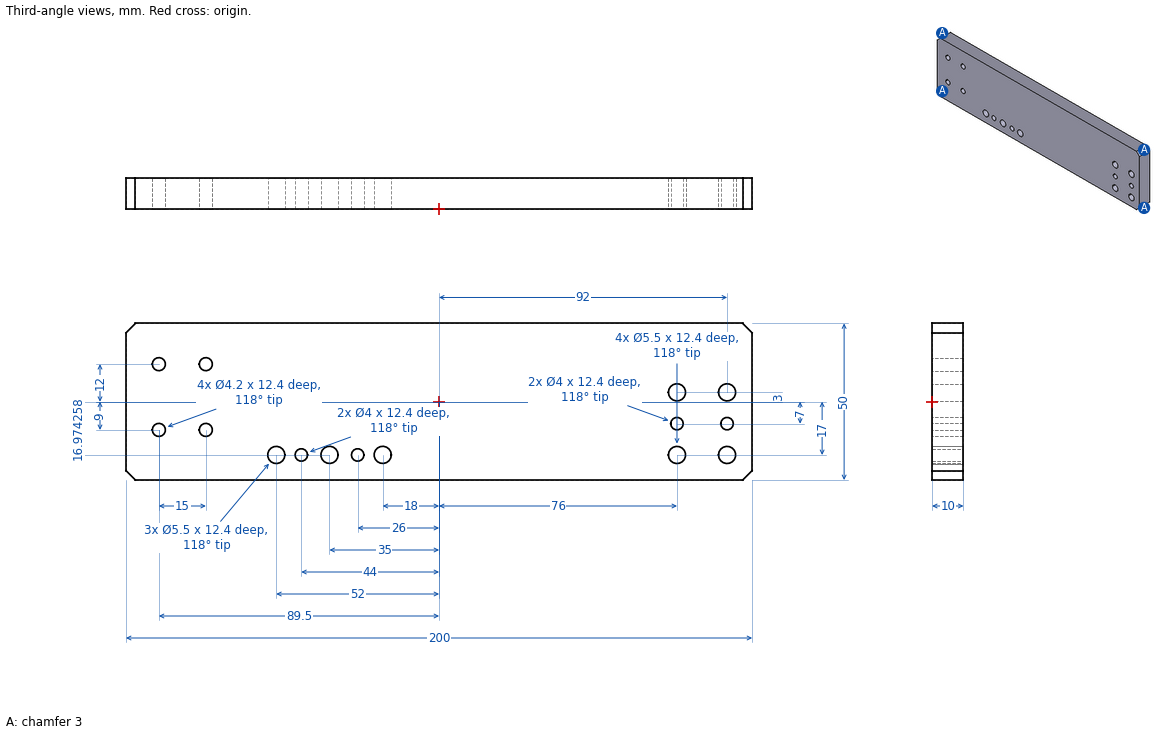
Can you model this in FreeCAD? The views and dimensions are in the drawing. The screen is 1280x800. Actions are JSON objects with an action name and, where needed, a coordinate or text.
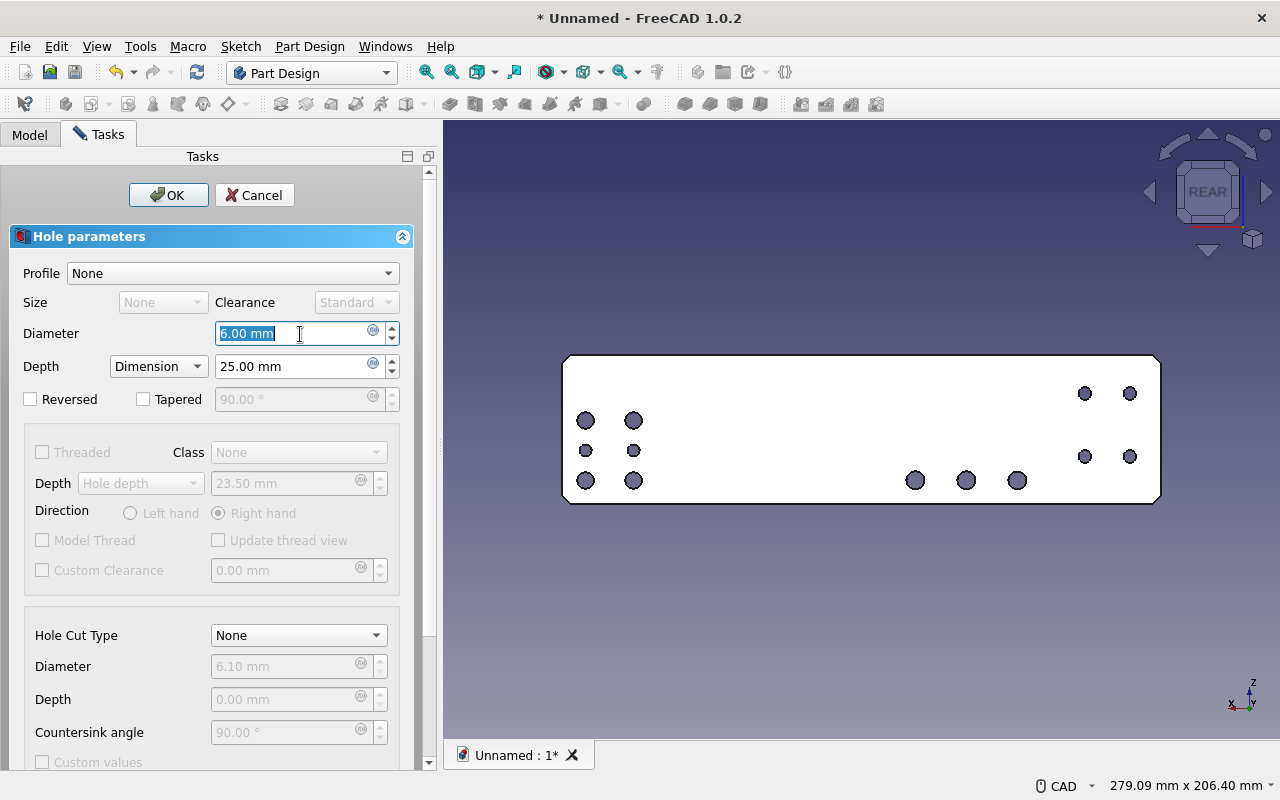
{"action": "type", "text": "5.5"}
{"action": "key", "text": "Tab"}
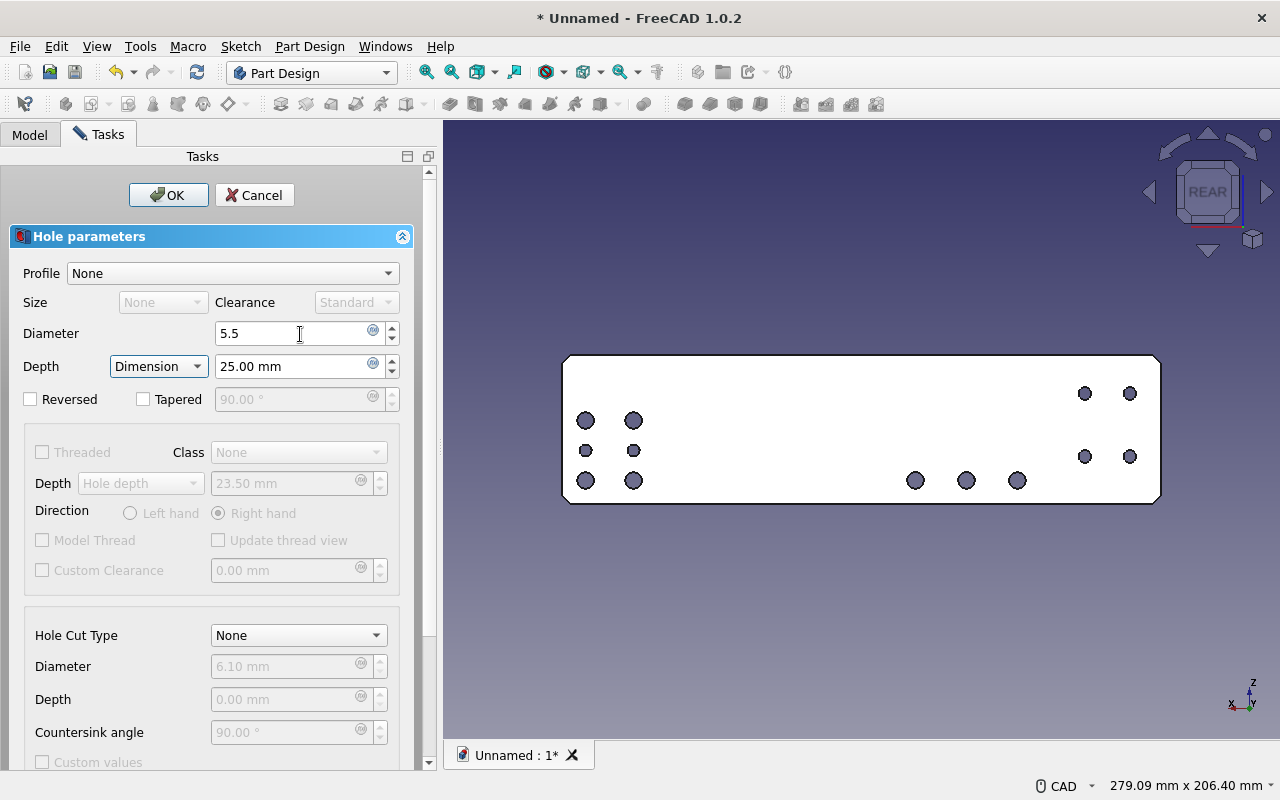
{"action": "triple_click", "coordinate": [300, 366]}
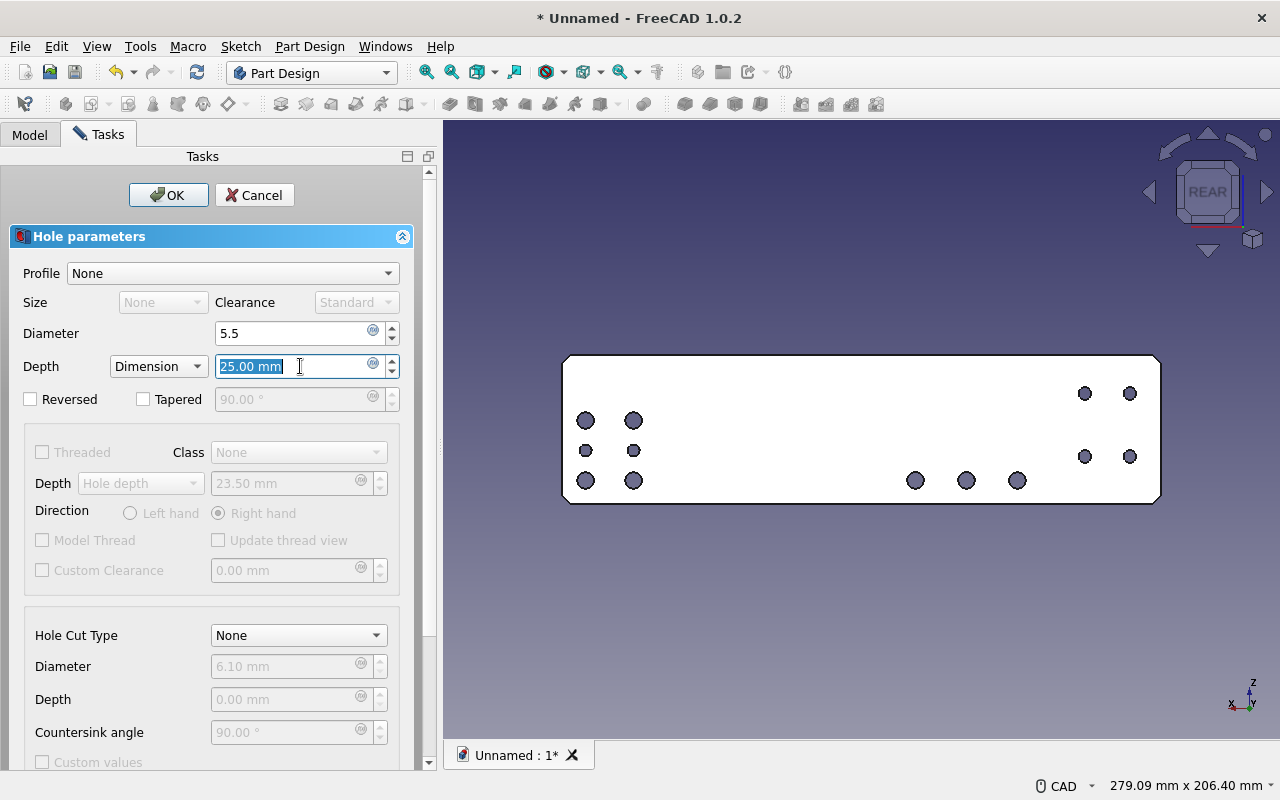
{"action": "type", "text": "12.4"}
{"action": "key", "text": "Tab"}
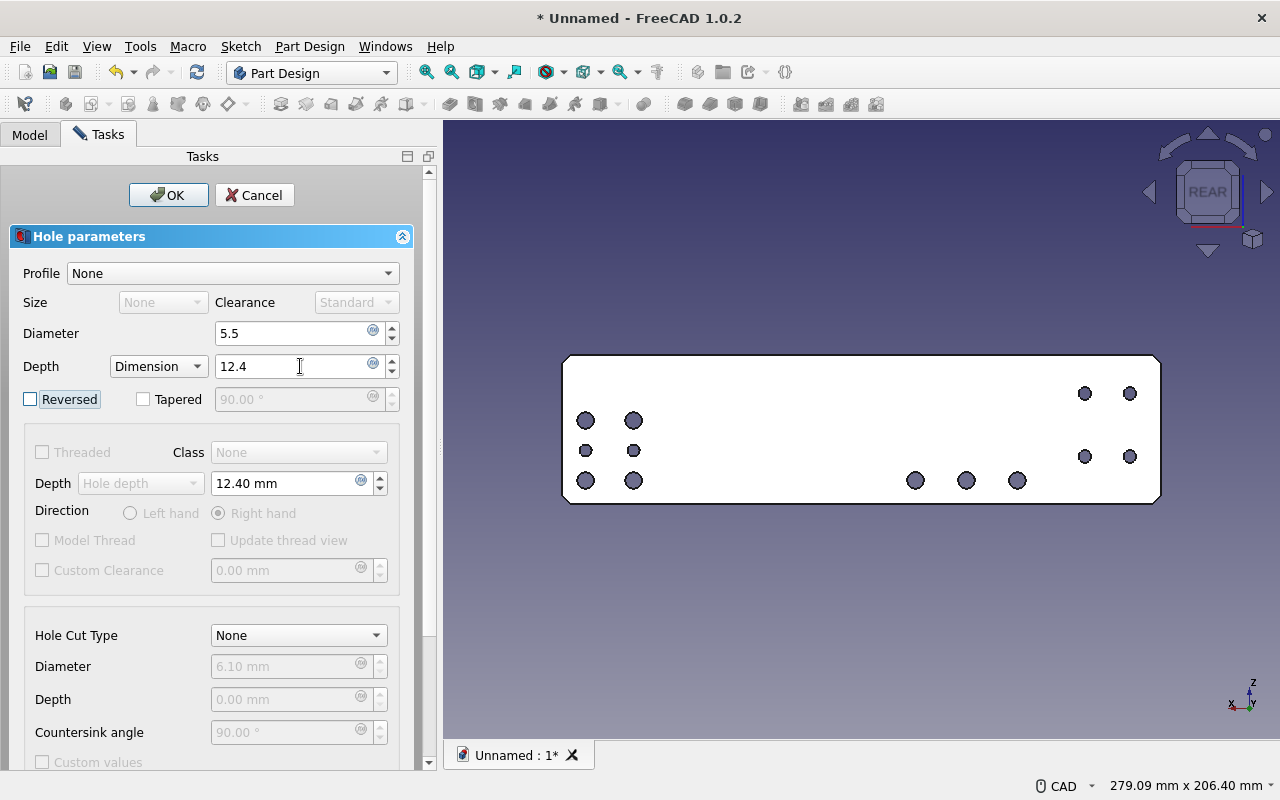
{"action": "left_click", "coordinate": [169, 195]}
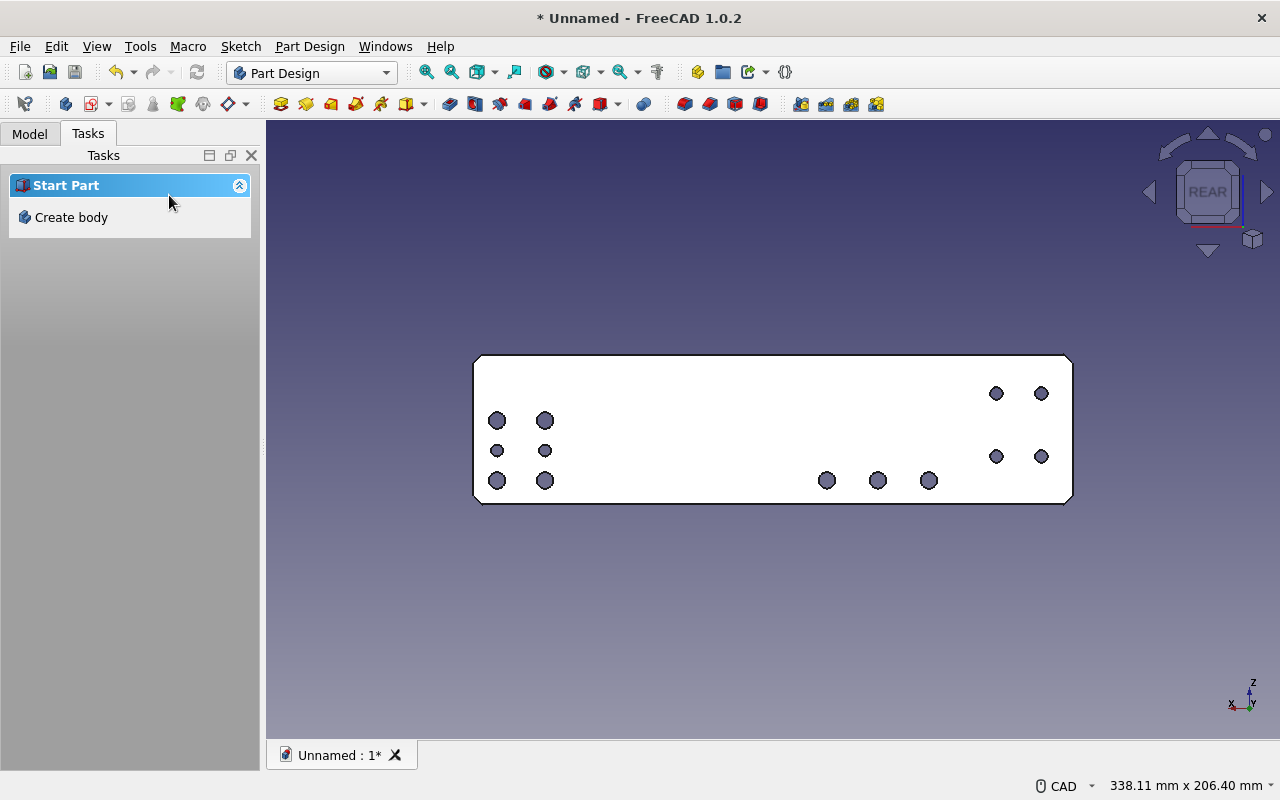
{"action": "left_click", "coordinate": [90, 104]}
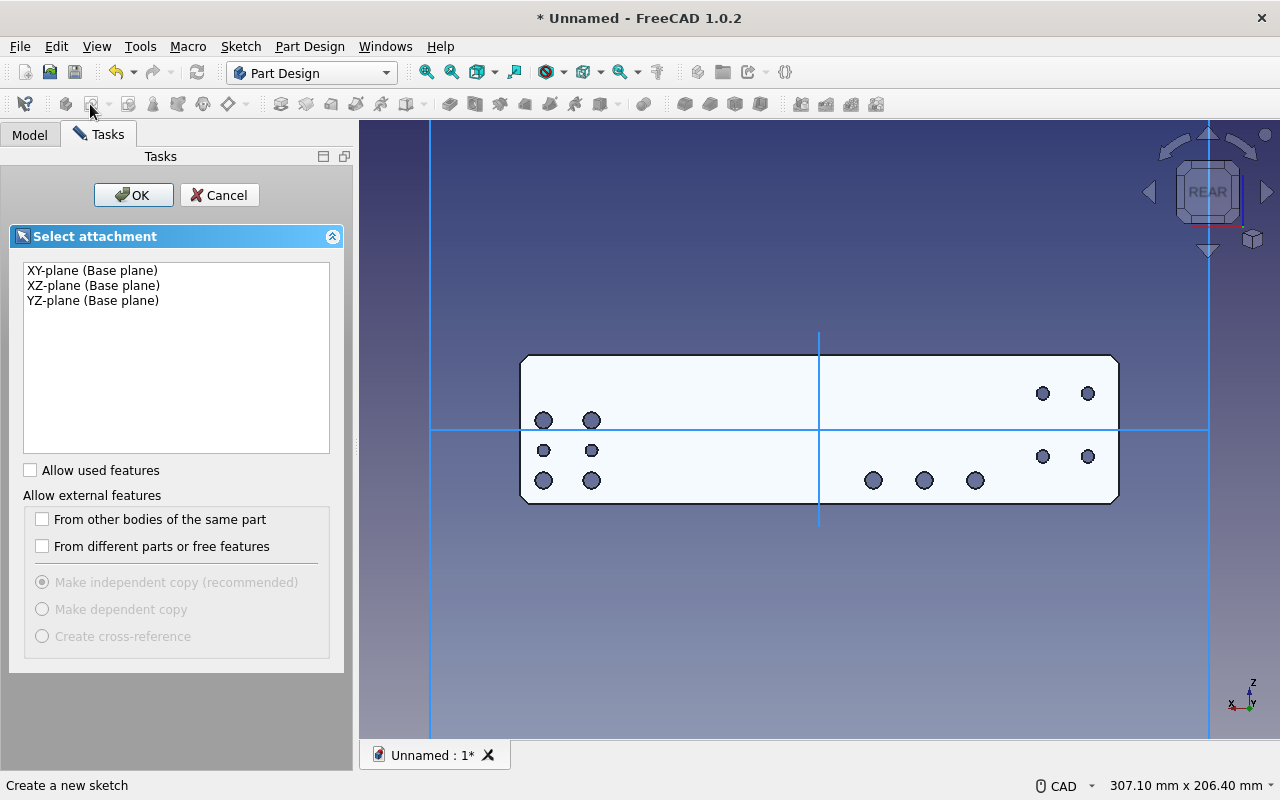
{"action": "left_click", "coordinate": [84, 286]}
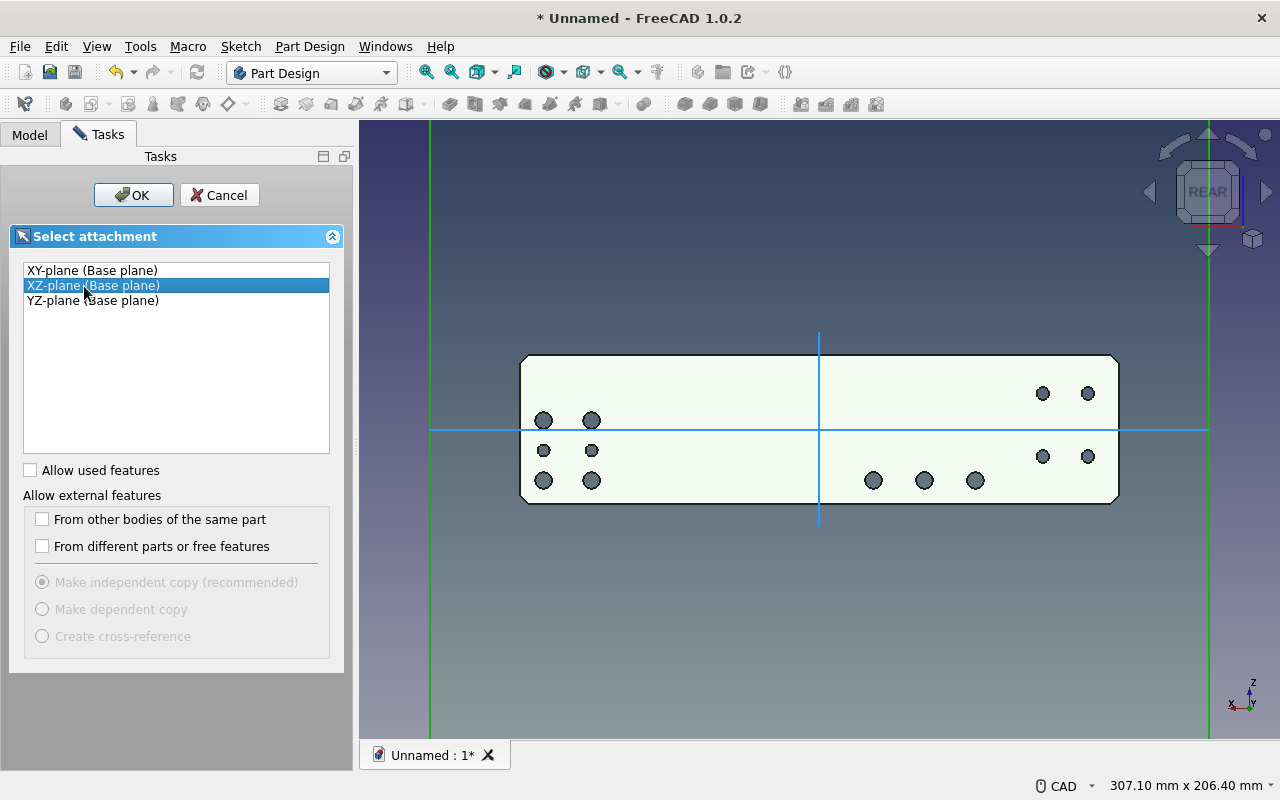
{"action": "left_click", "coordinate": [134, 195]}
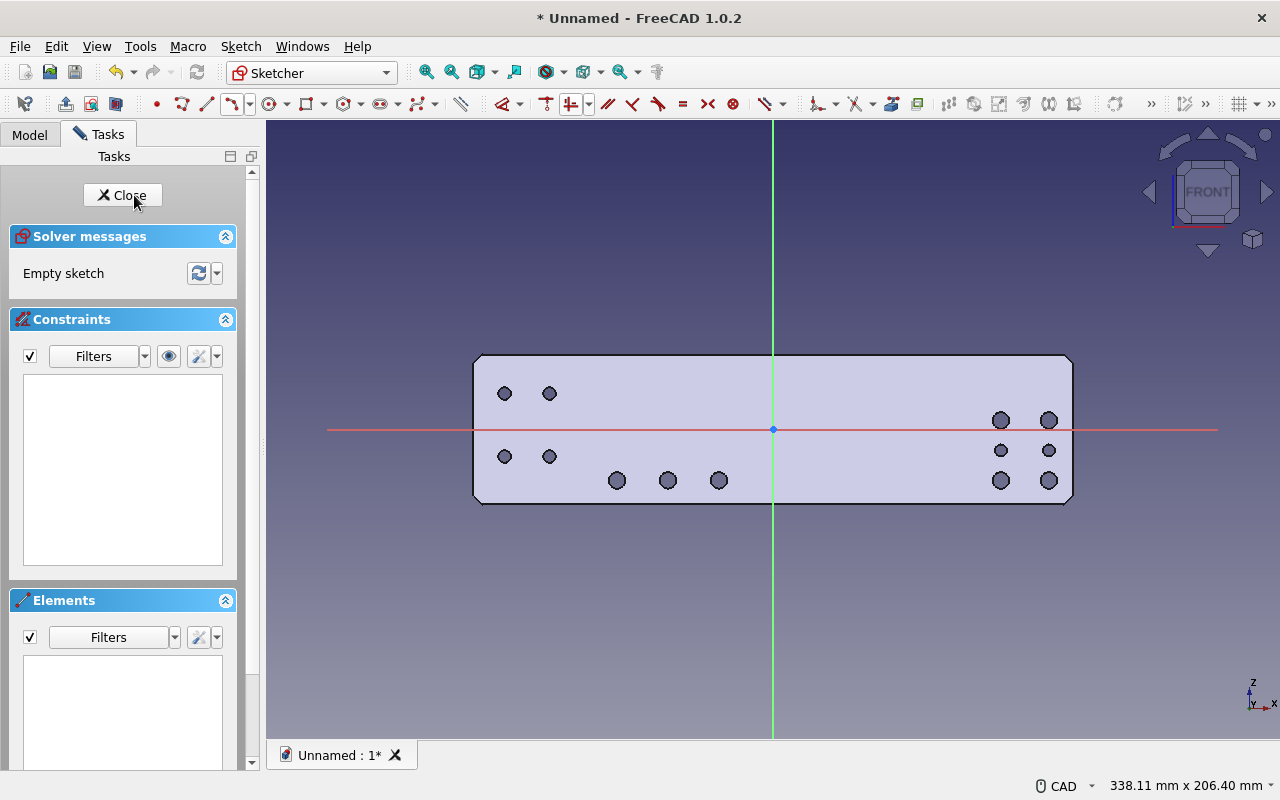
{"action": "scroll", "coordinate": [704, 467], "scroll_direction": "up", "scroll_amount": 7}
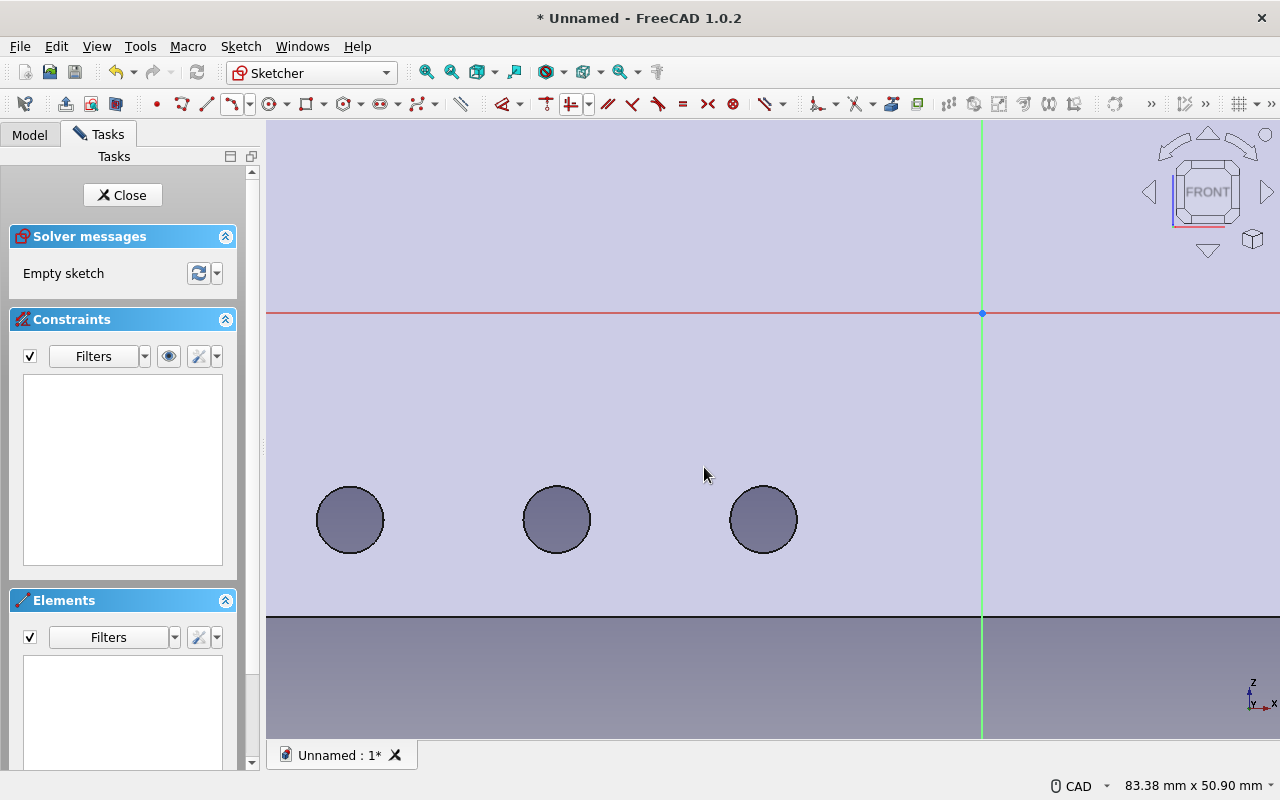
{"action": "left_click", "coordinate": [268, 104]}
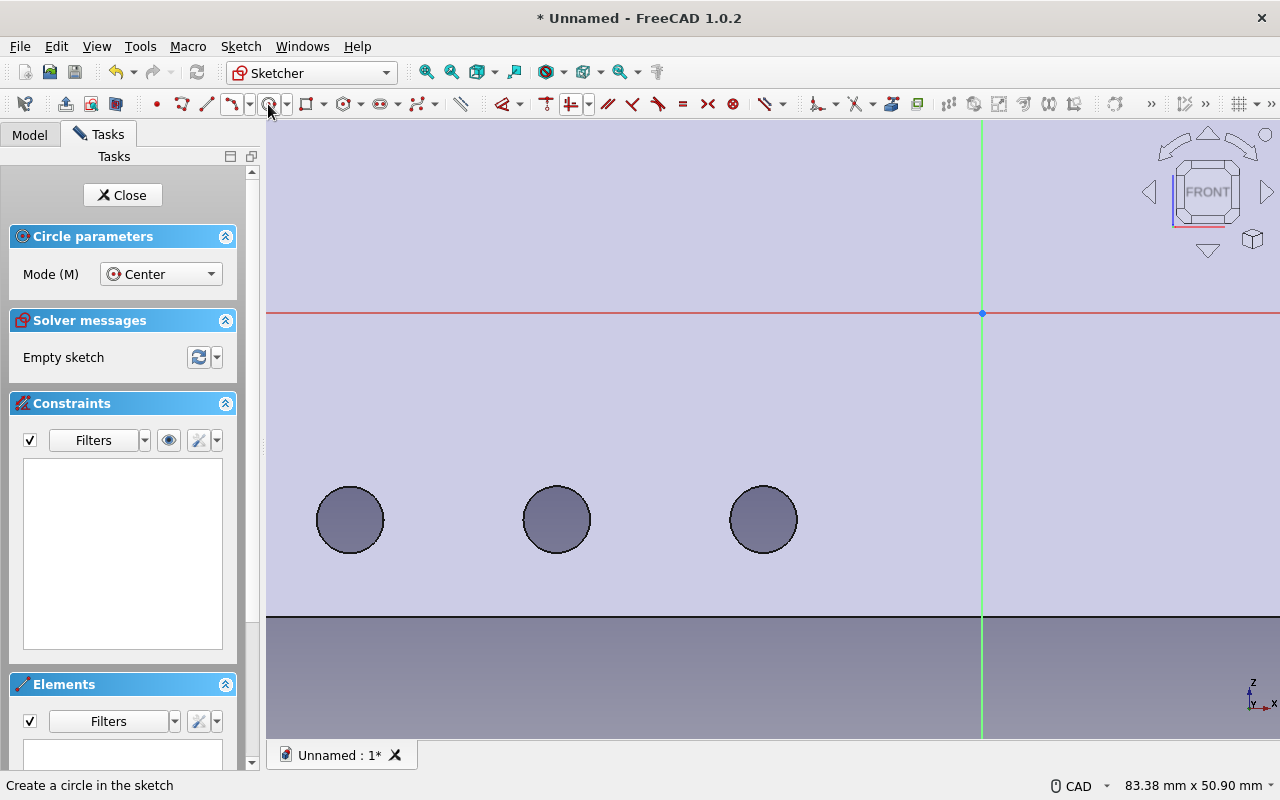
{"action": "left_click", "coordinate": [447, 520]}
{"action": "left_click", "coordinate": [465, 503]}